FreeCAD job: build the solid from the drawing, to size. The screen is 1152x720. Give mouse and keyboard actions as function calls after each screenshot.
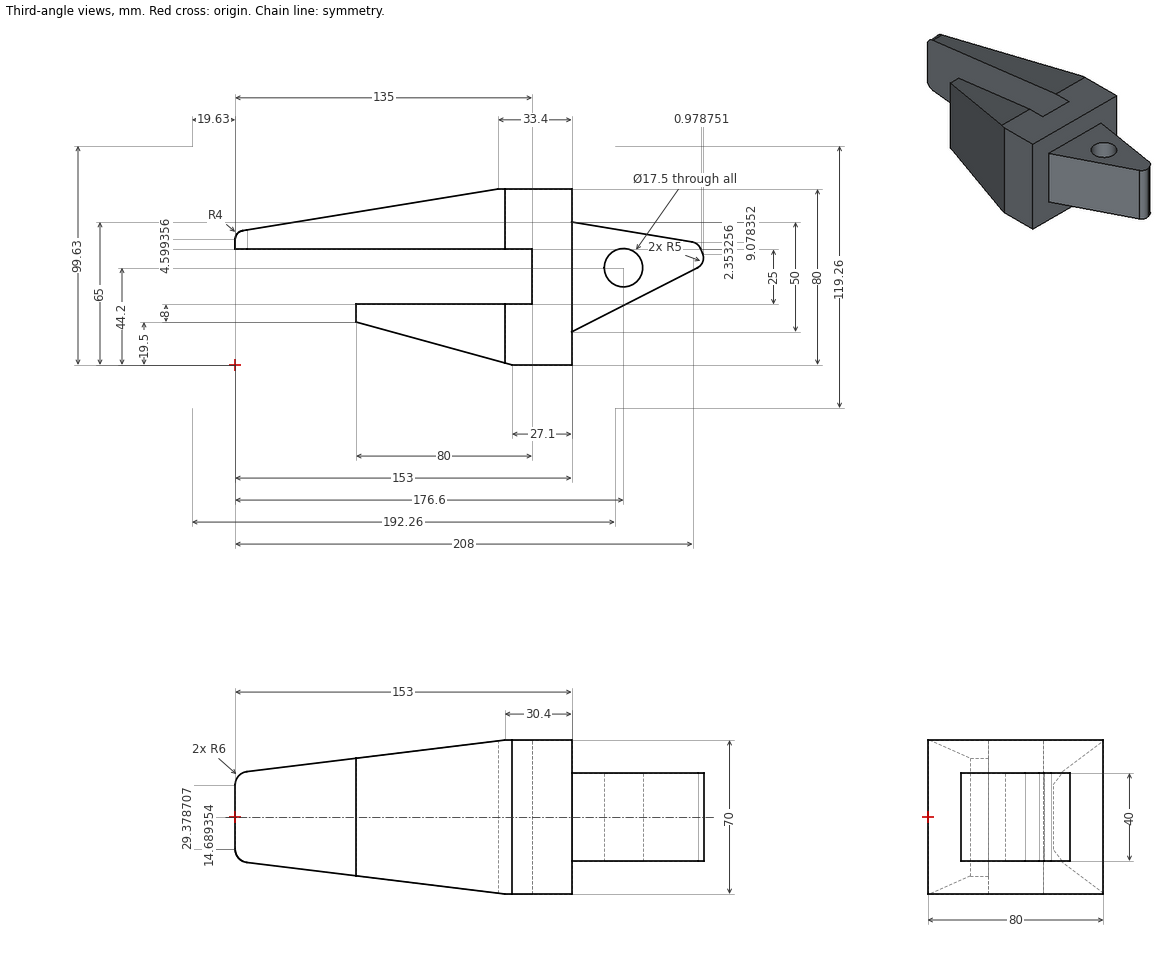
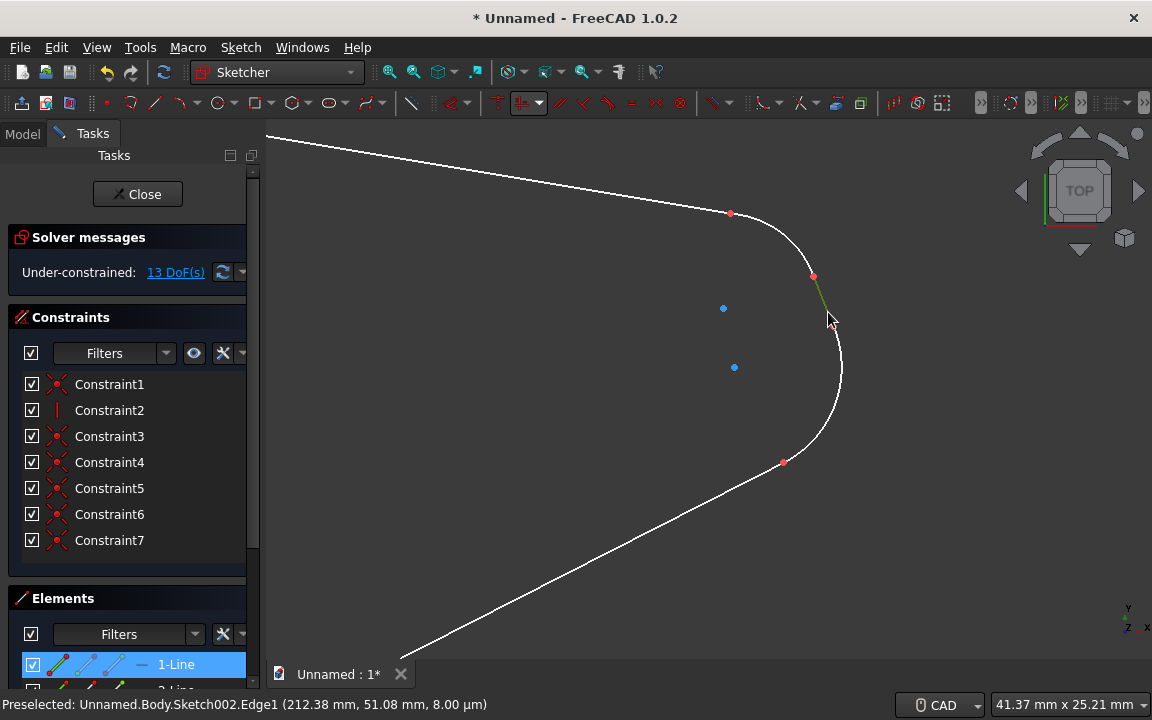
click(797, 248)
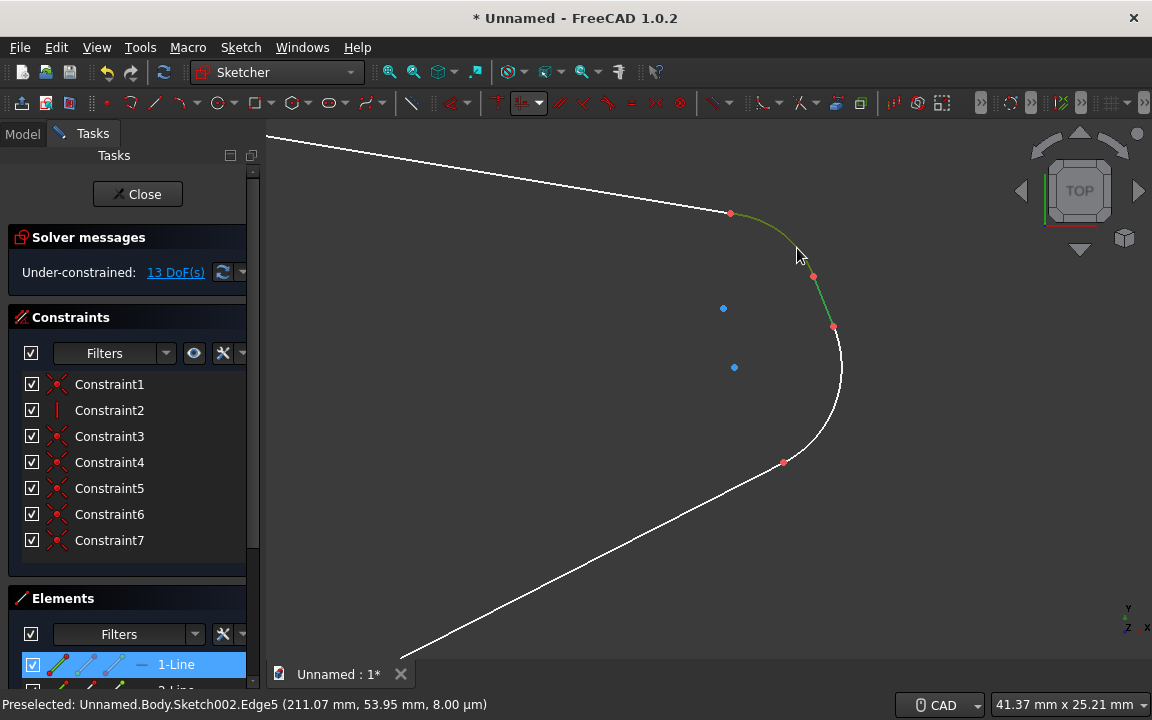
key(t)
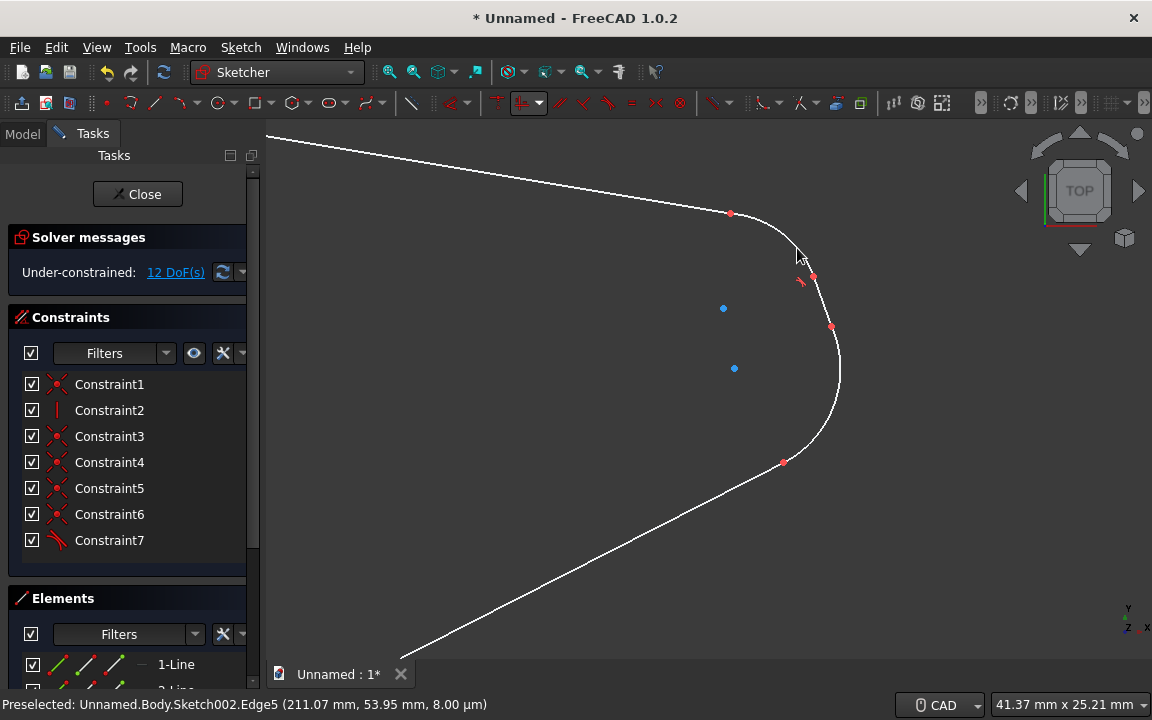
click(826, 312)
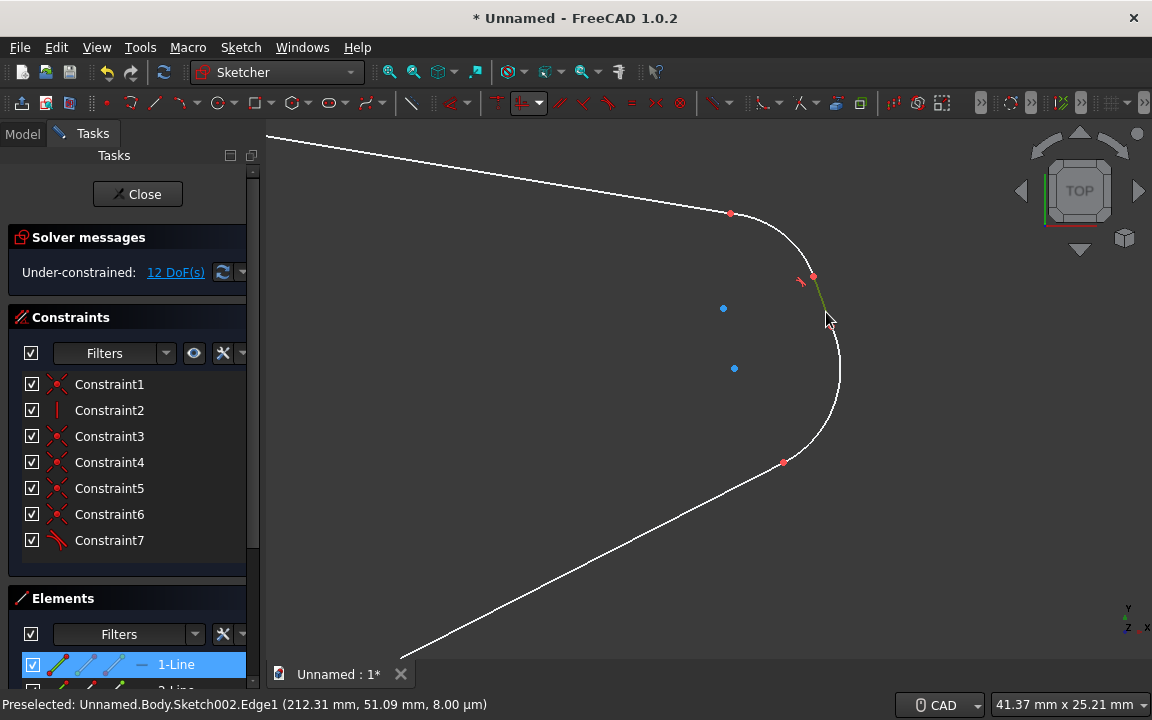
click(820, 432)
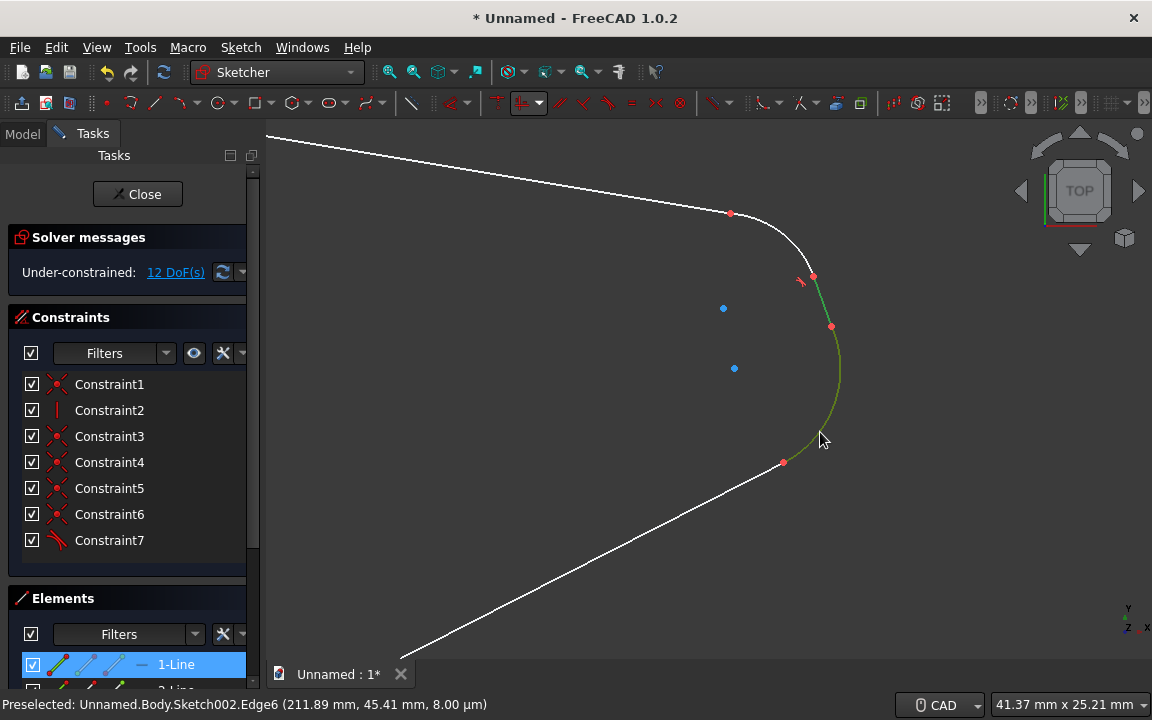
click(608, 104)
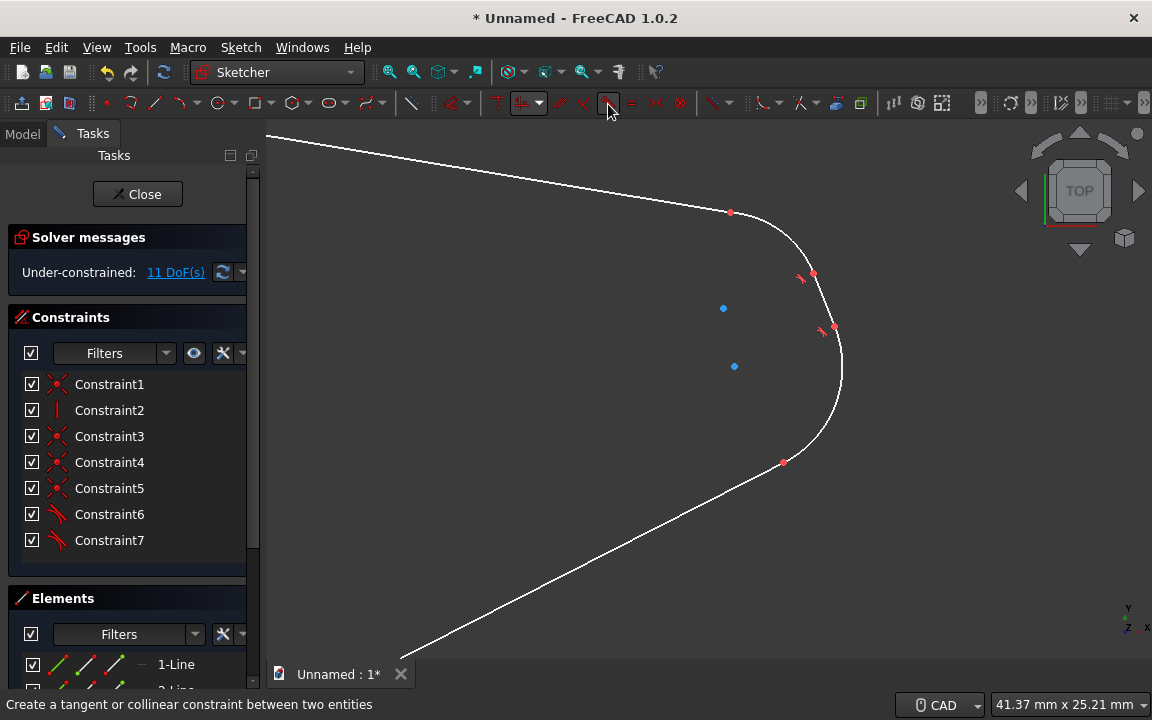
click(378, 154)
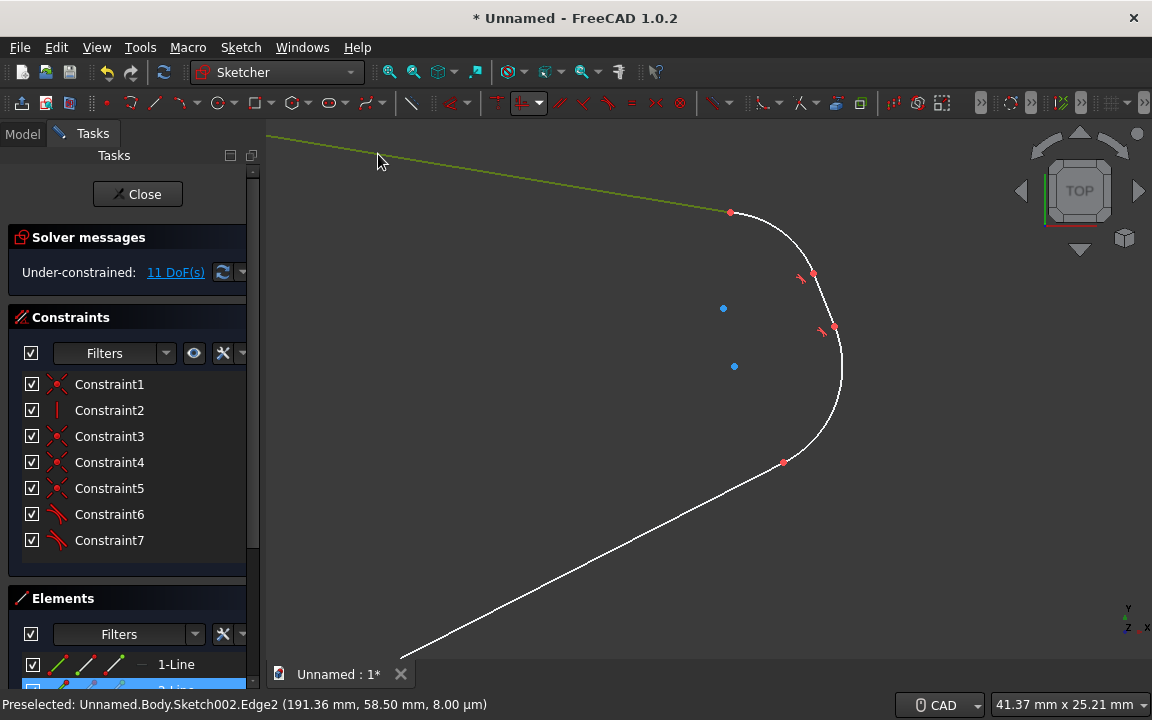
click(797, 246)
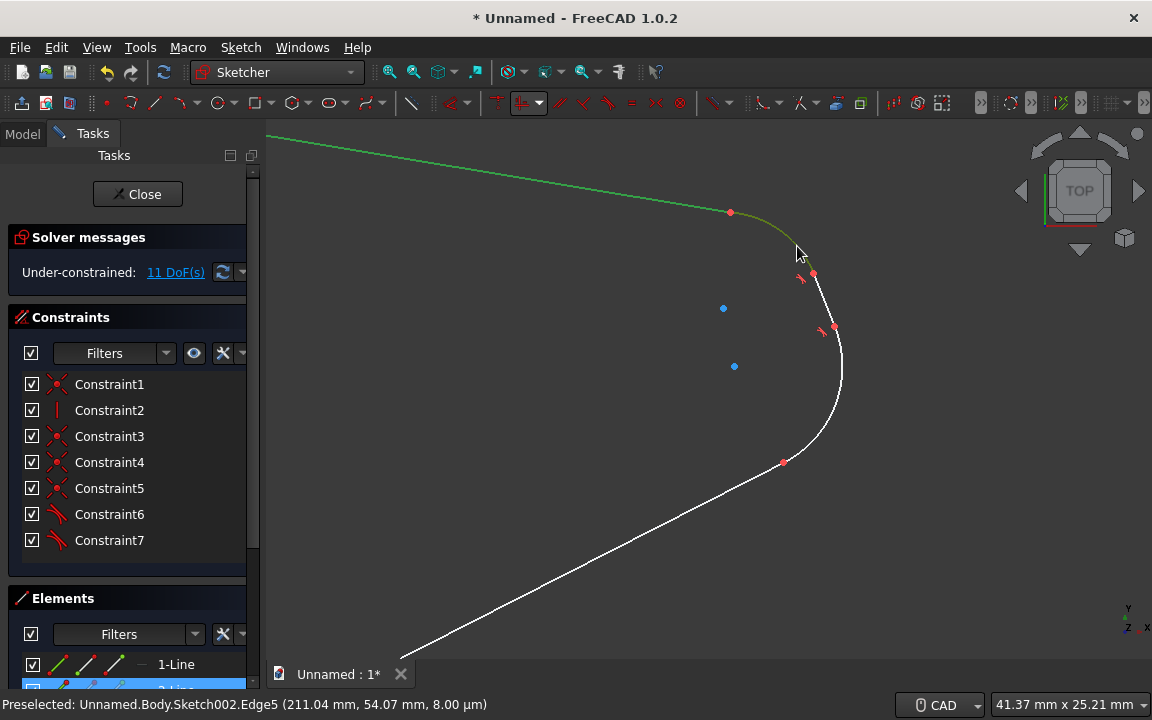
click(608, 104)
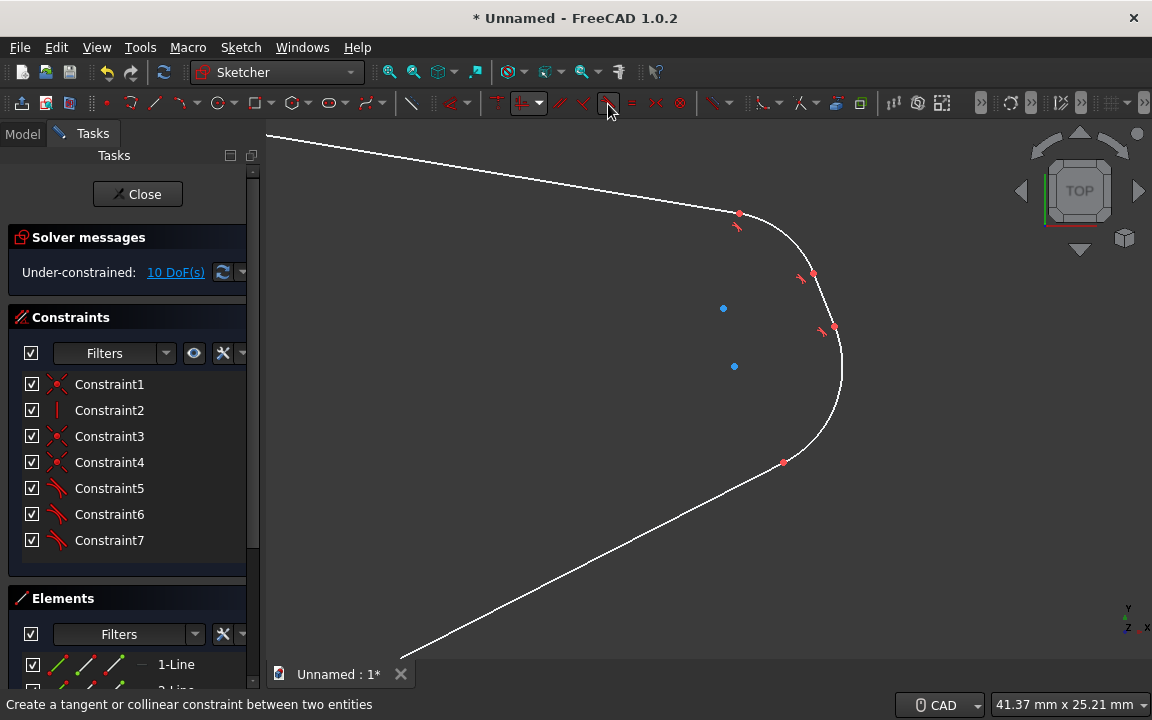
click(538, 588)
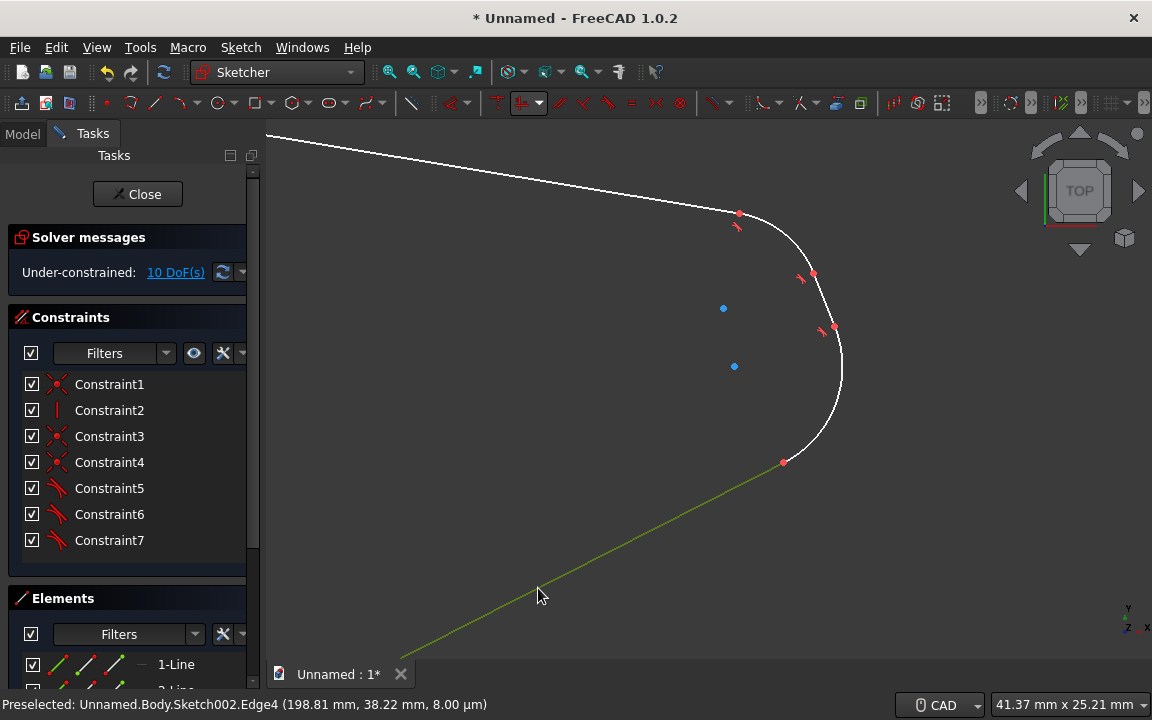
click(820, 432)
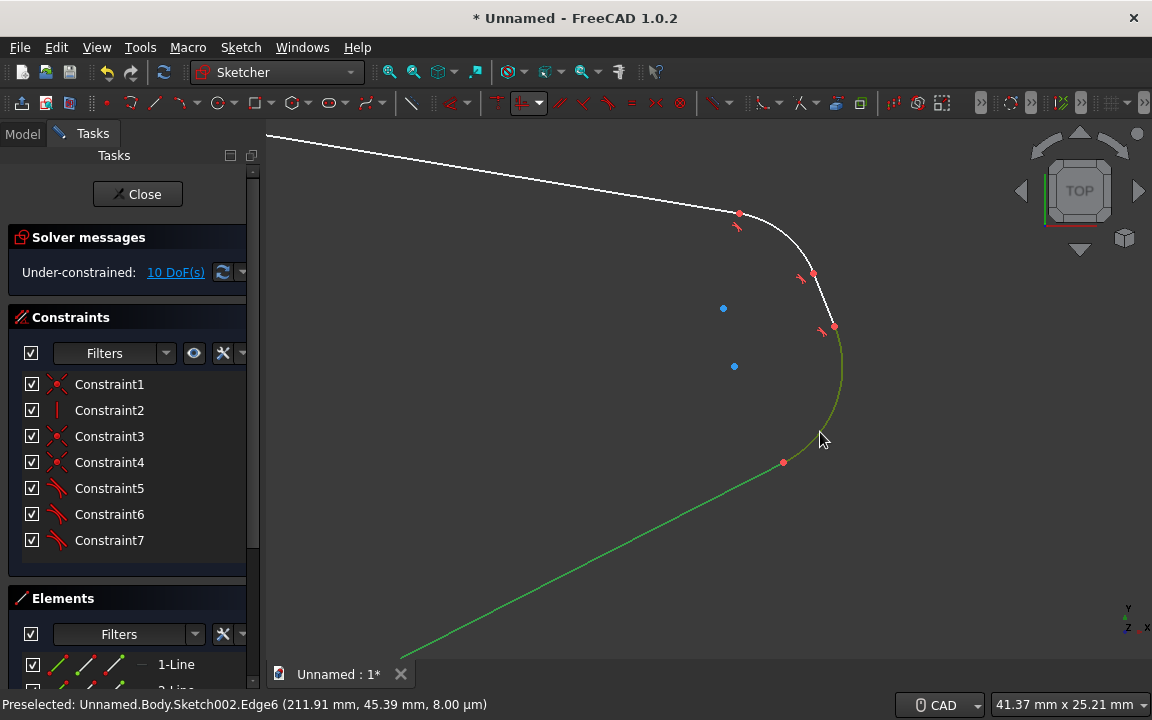
click(608, 104)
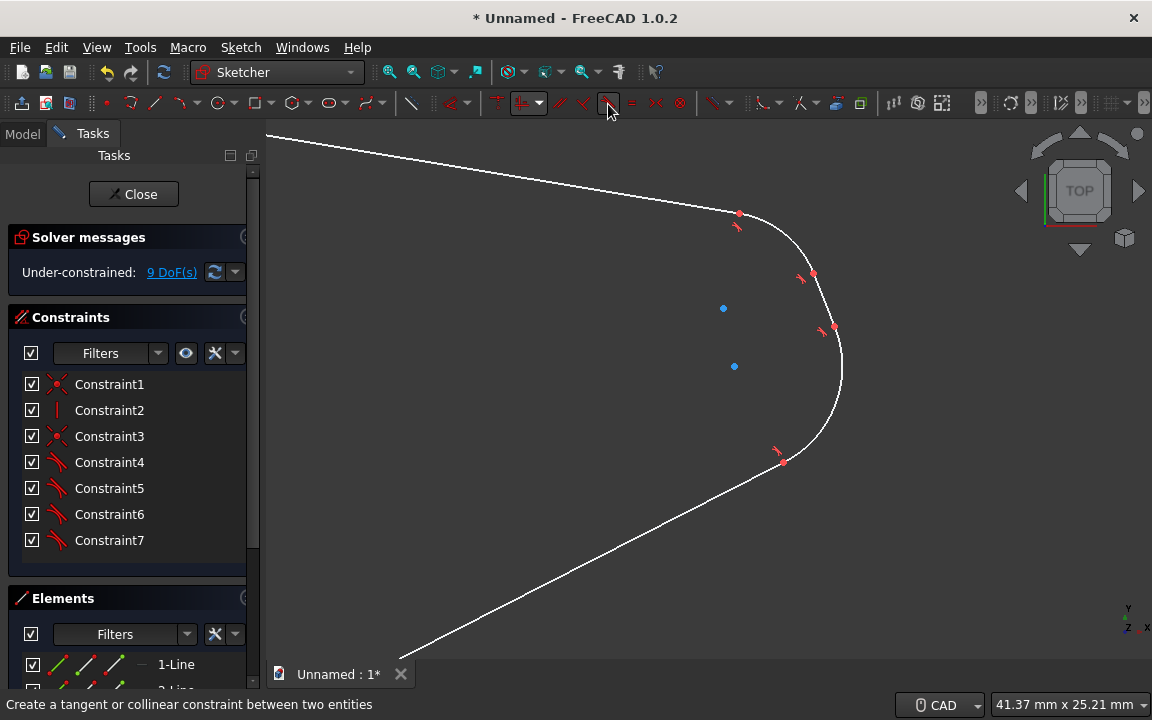
click(798, 248)